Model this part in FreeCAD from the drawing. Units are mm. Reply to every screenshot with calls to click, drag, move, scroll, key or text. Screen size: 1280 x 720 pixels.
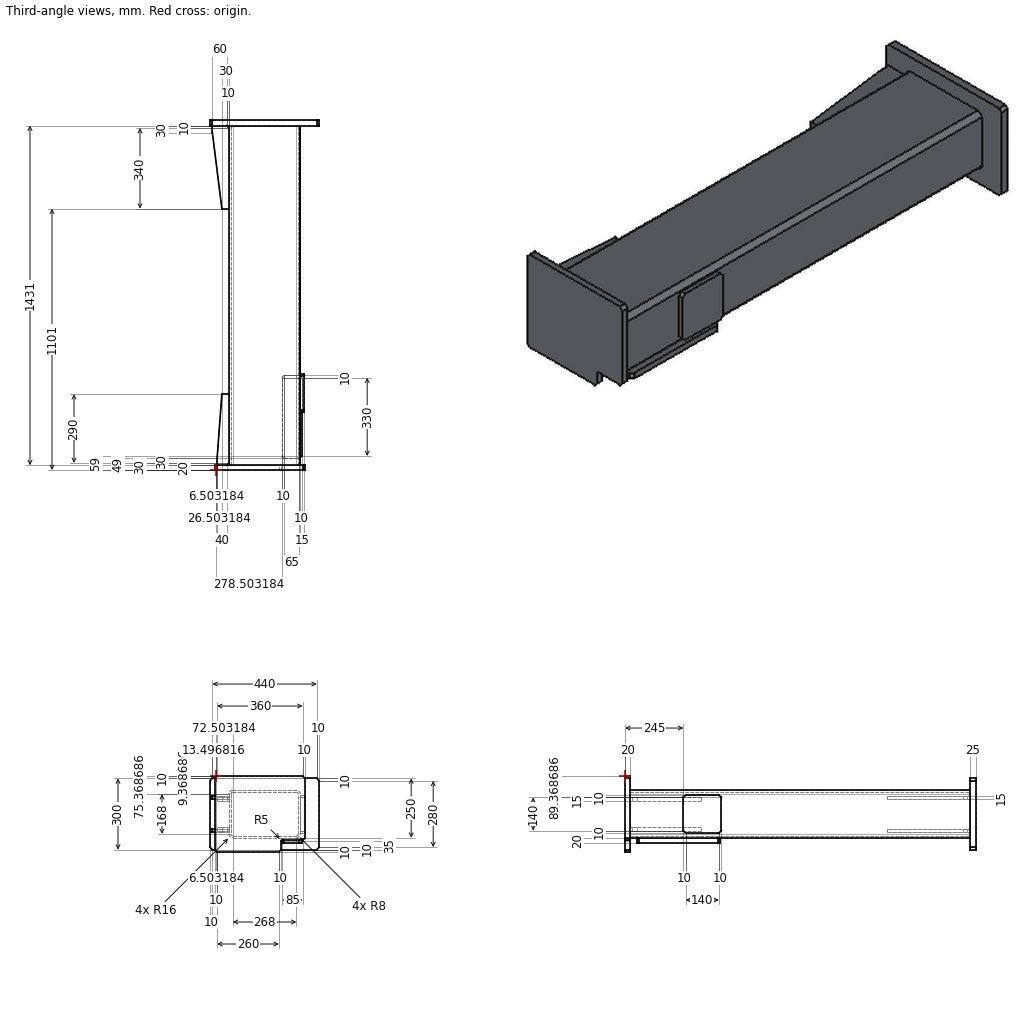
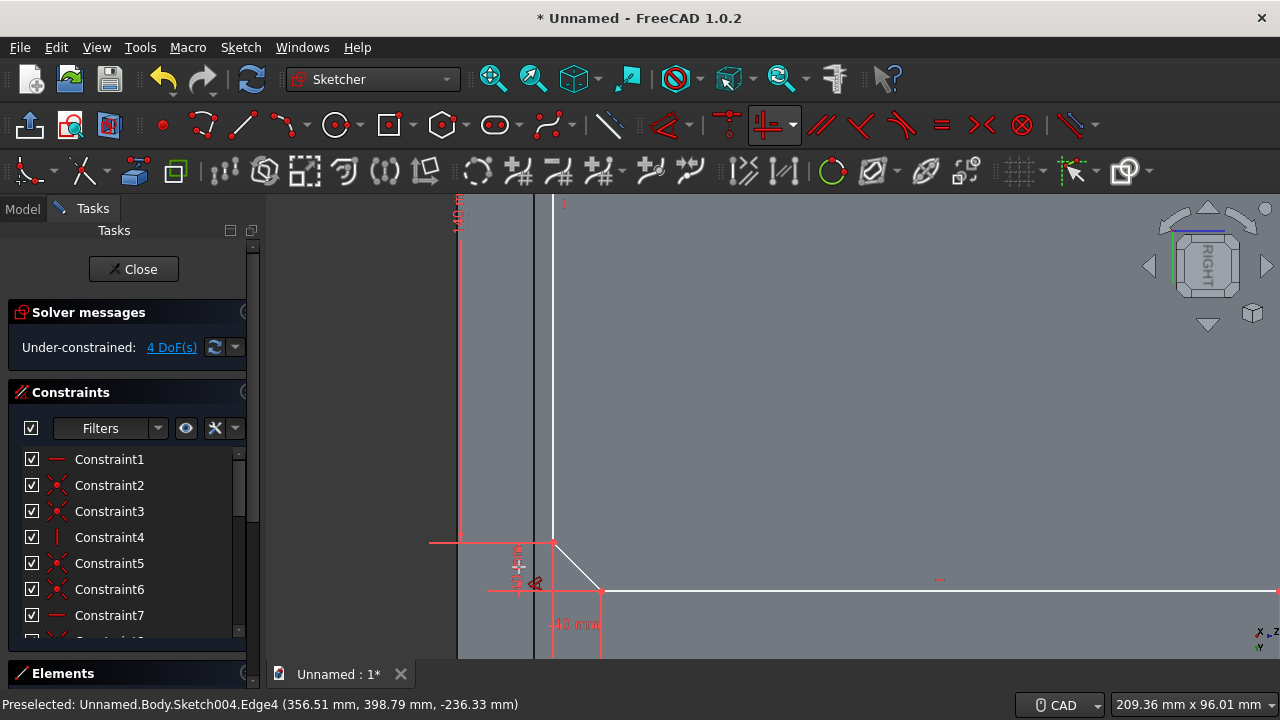
scroll(567, 558, down, 5)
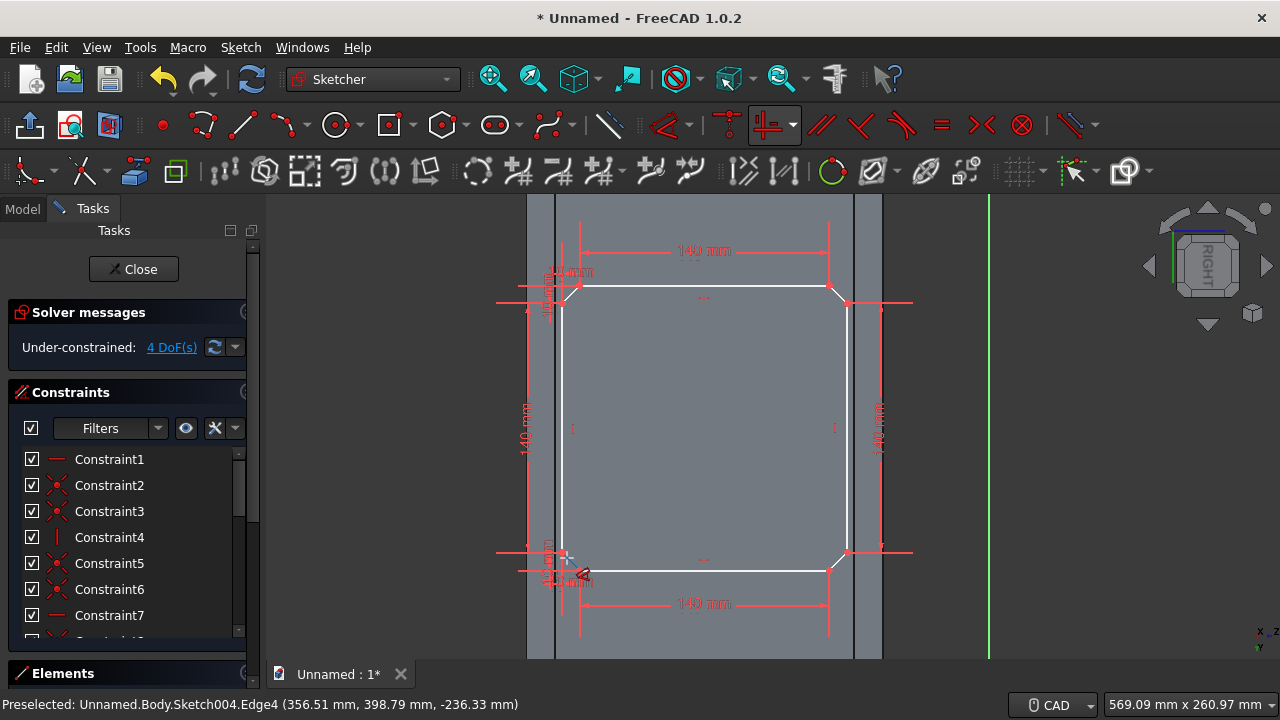
scroll(835, 565, up, 5)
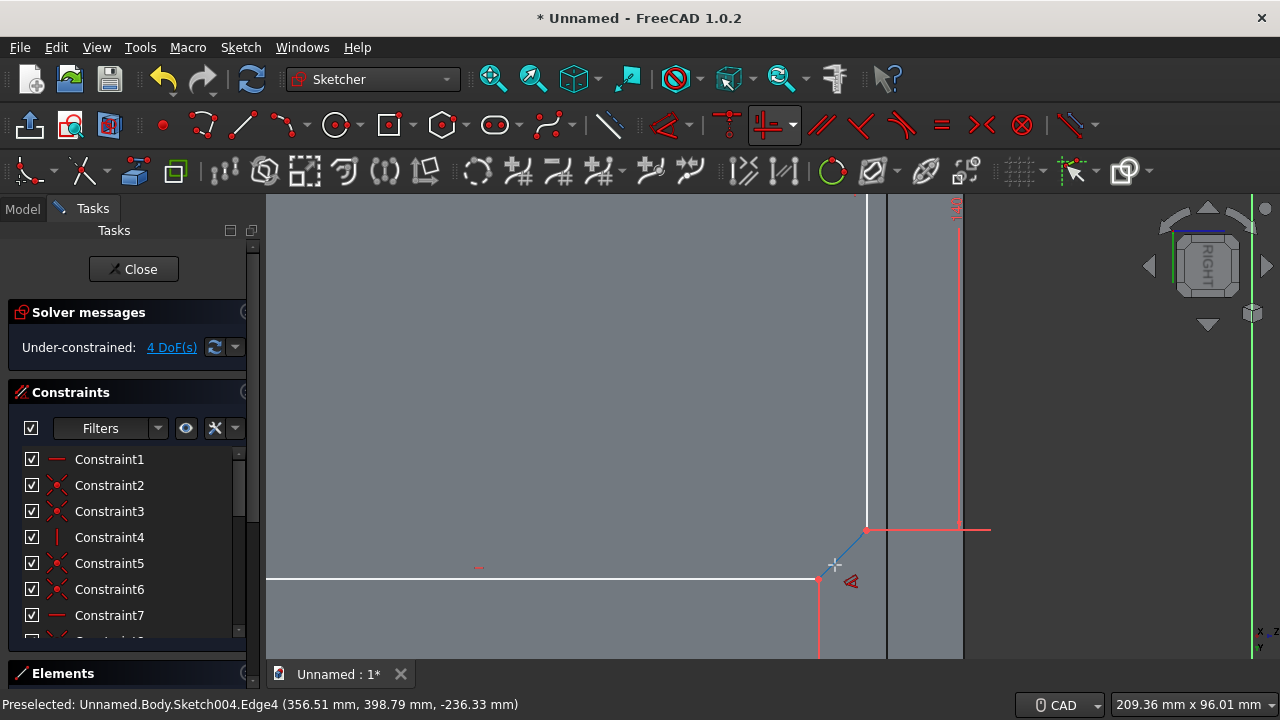
click(833, 564)
click(843, 613)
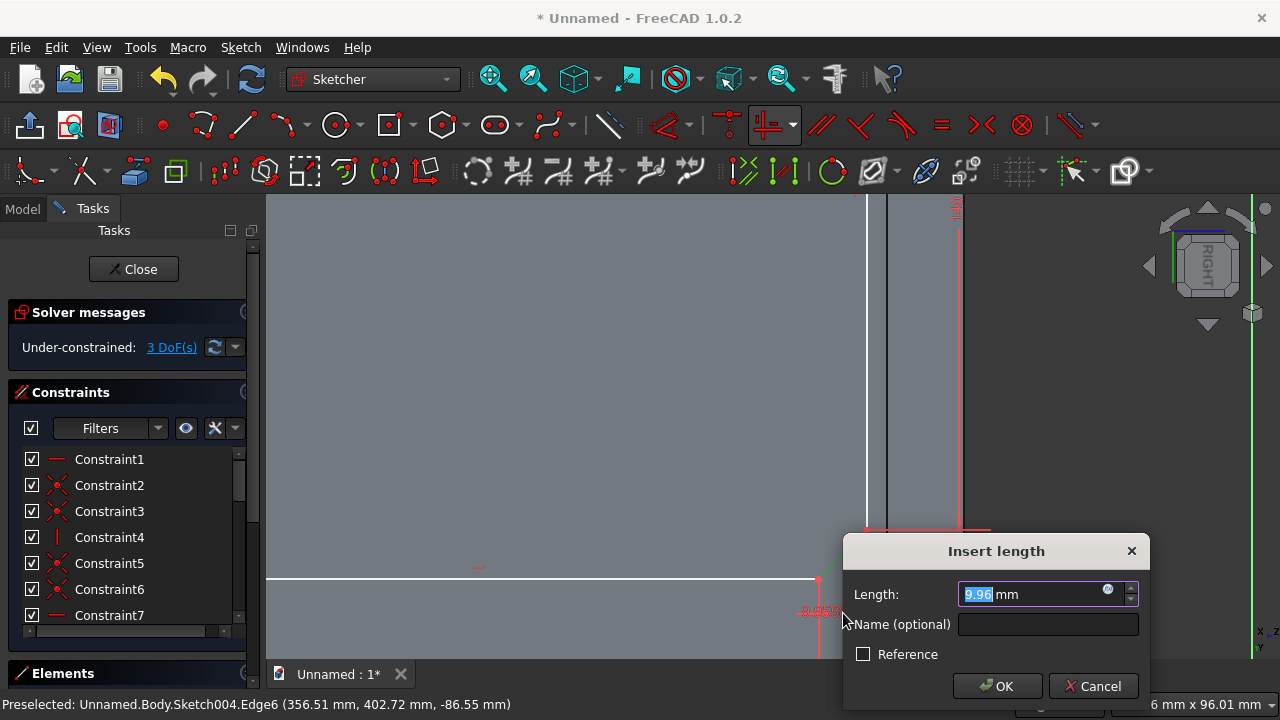
text(10)
key(Return)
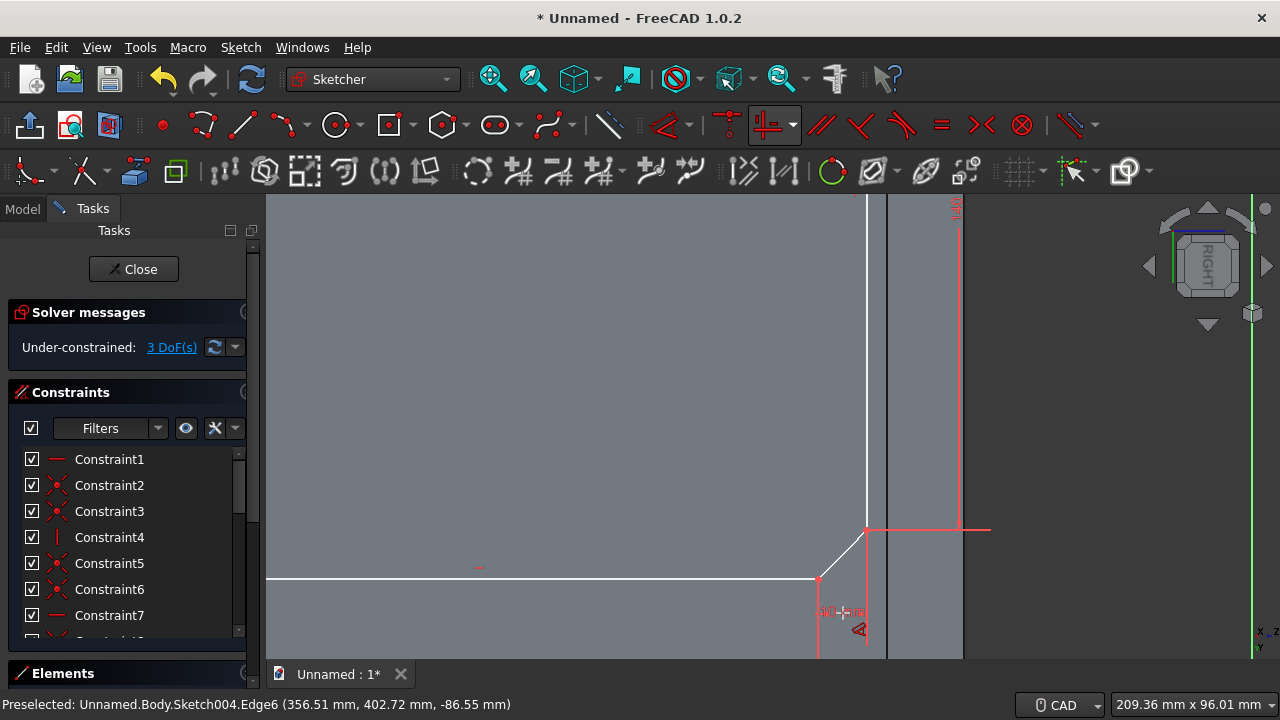
click(833, 564)
click(901, 555)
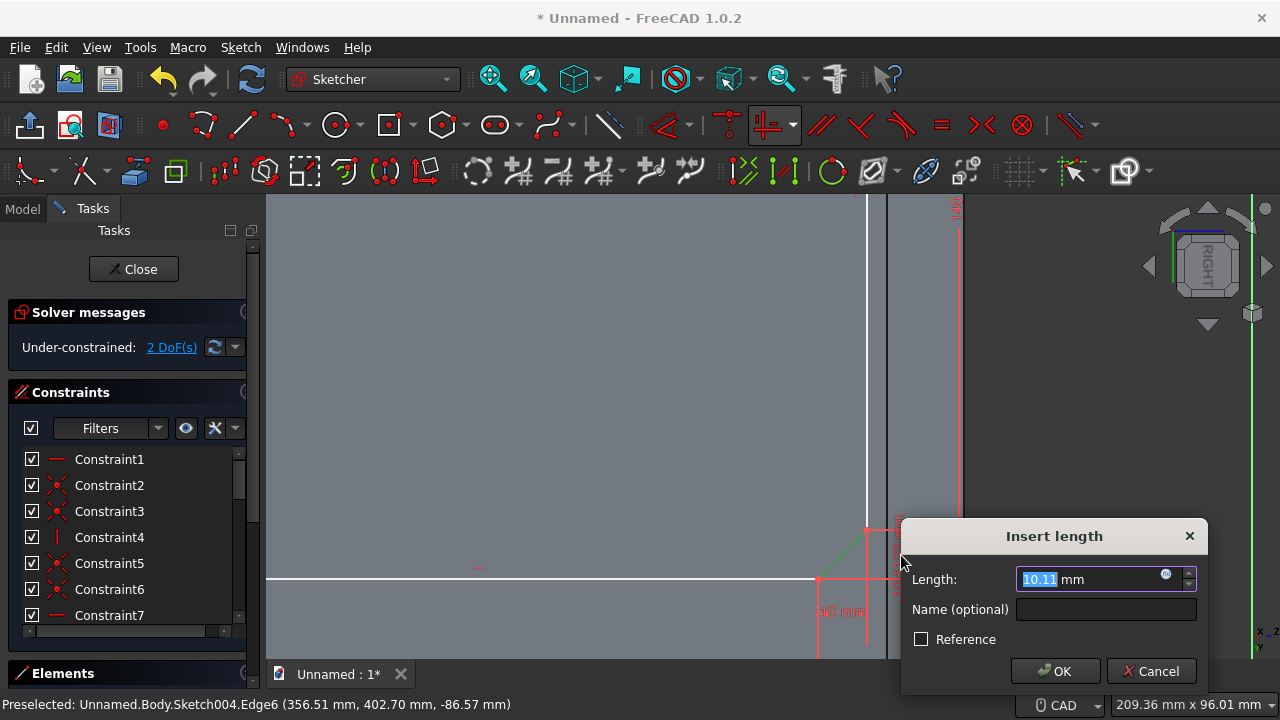
text(10)
key(Return)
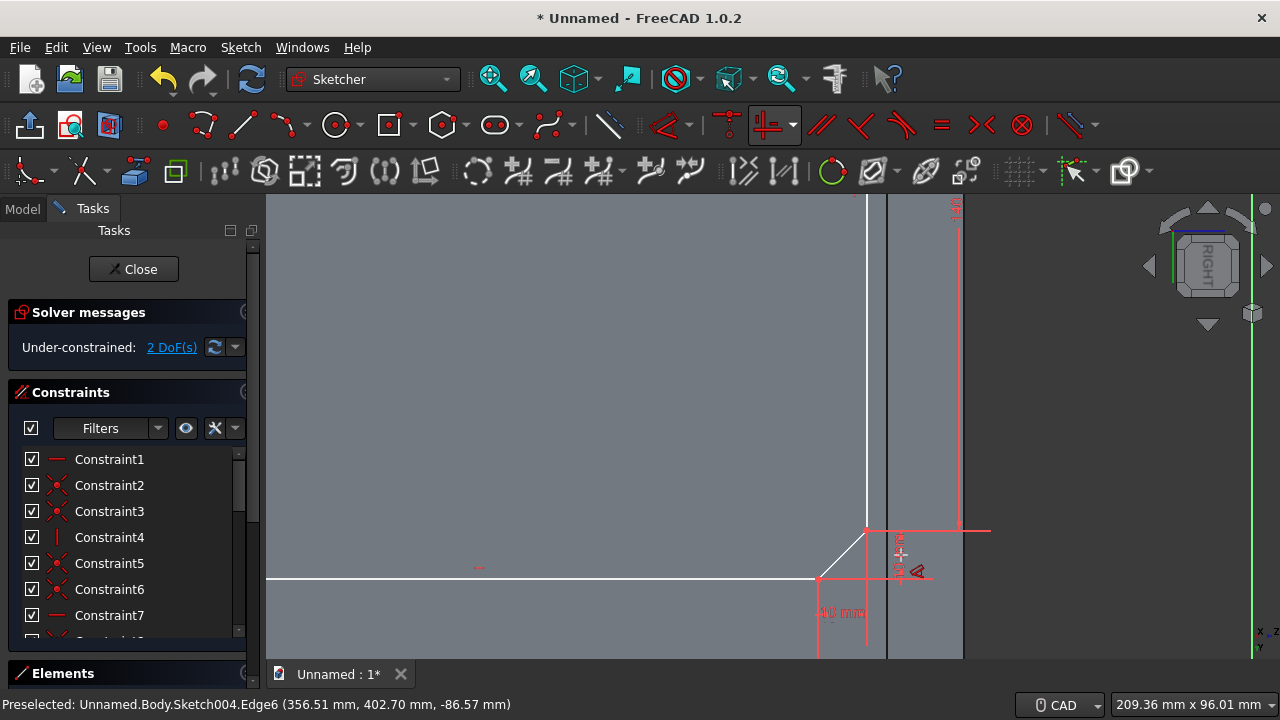
scroll(835, 565, down, 5)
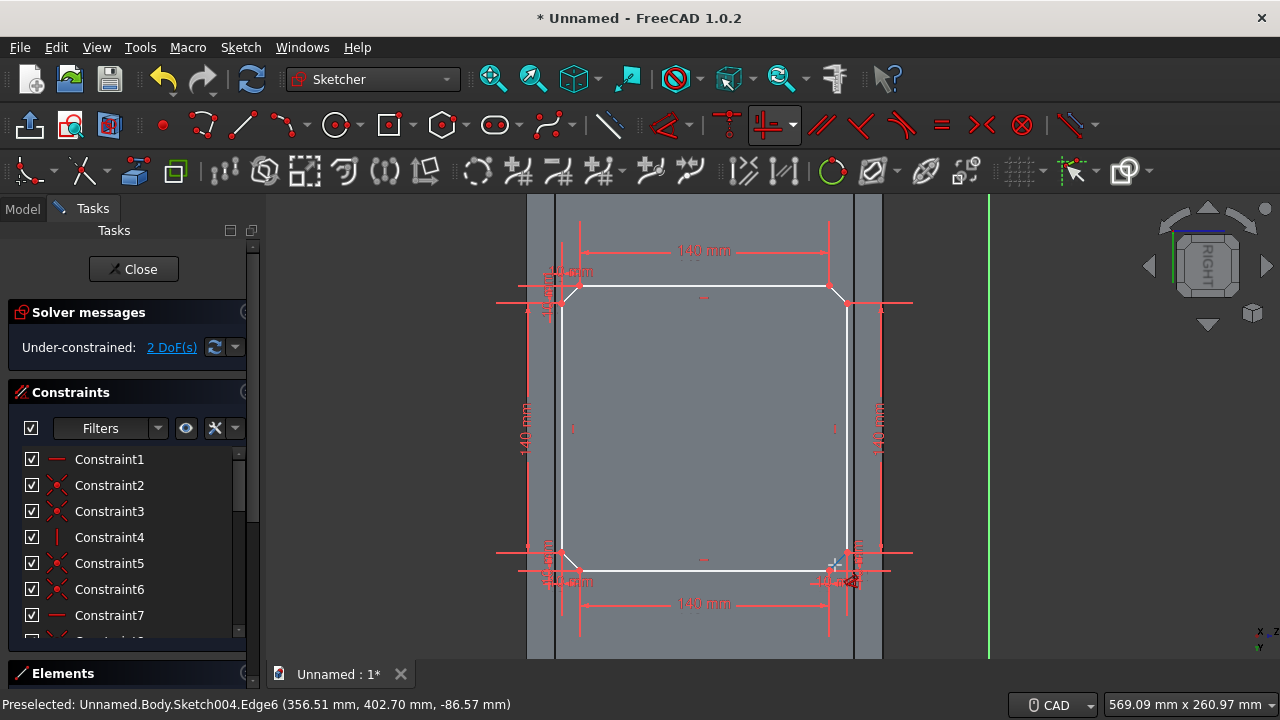
click(829, 286)
click(1023, 254)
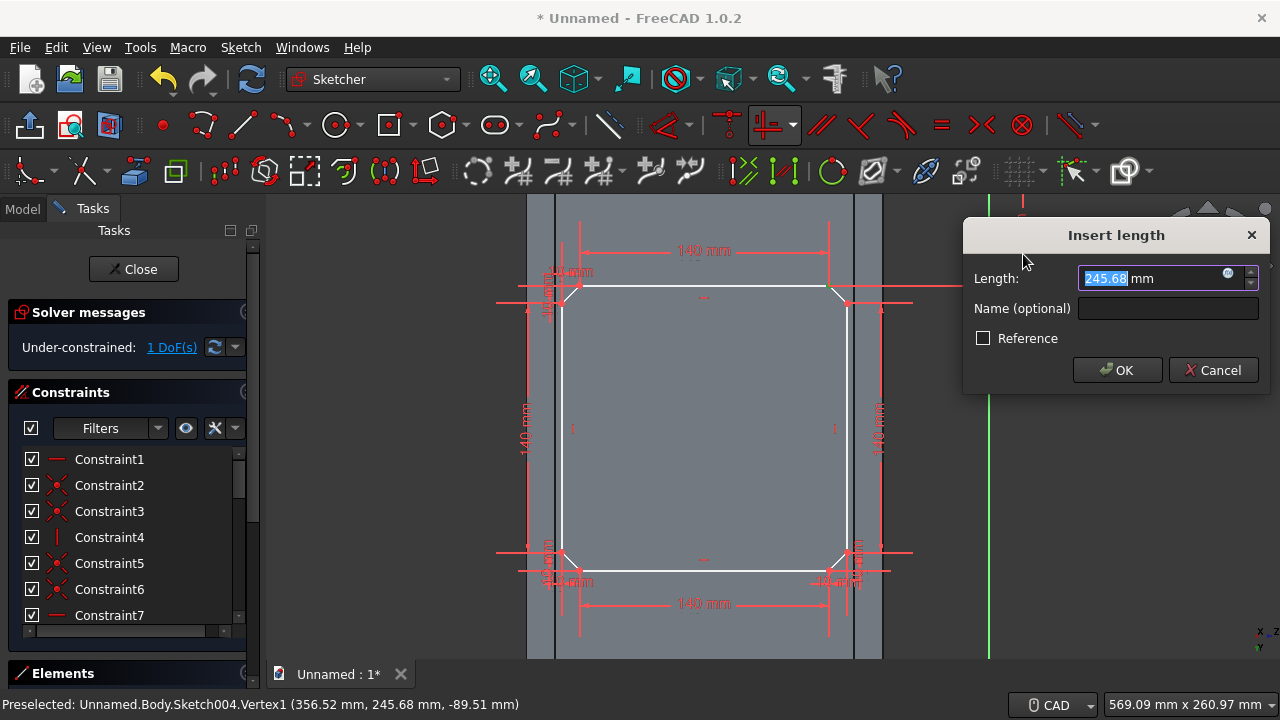
text(245)
key(Return)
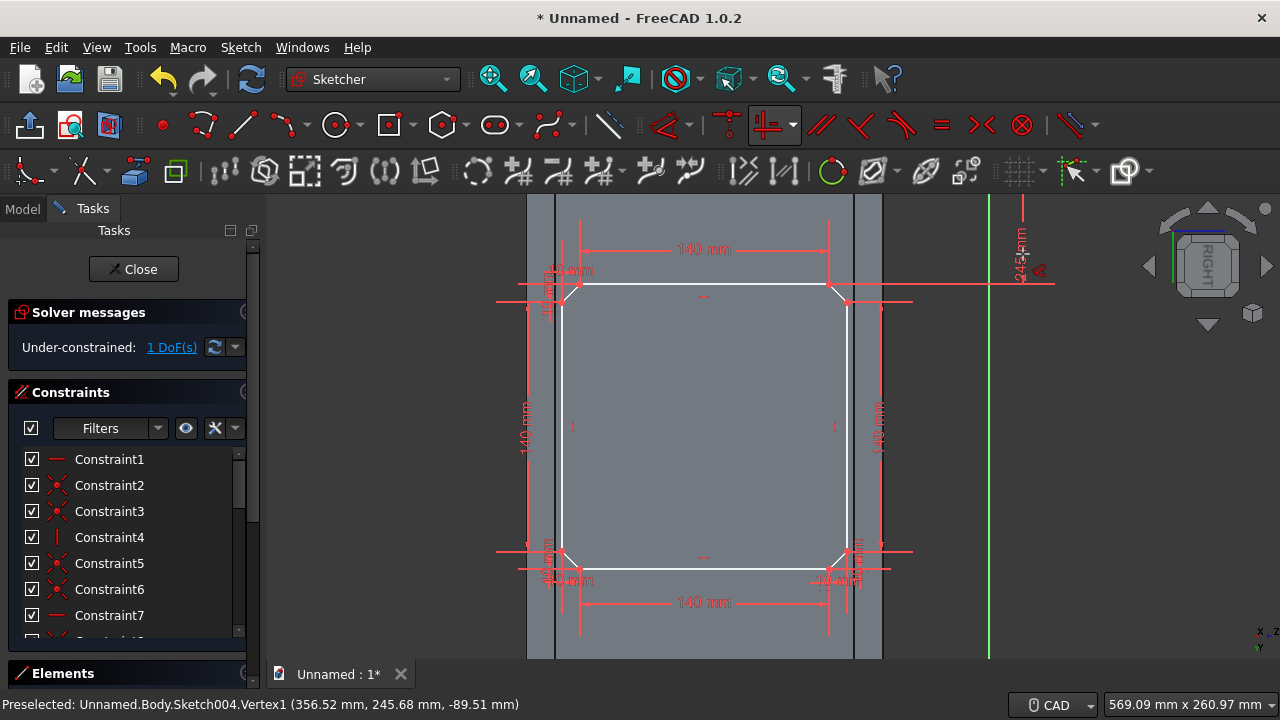
click(829, 284)
click(909, 318)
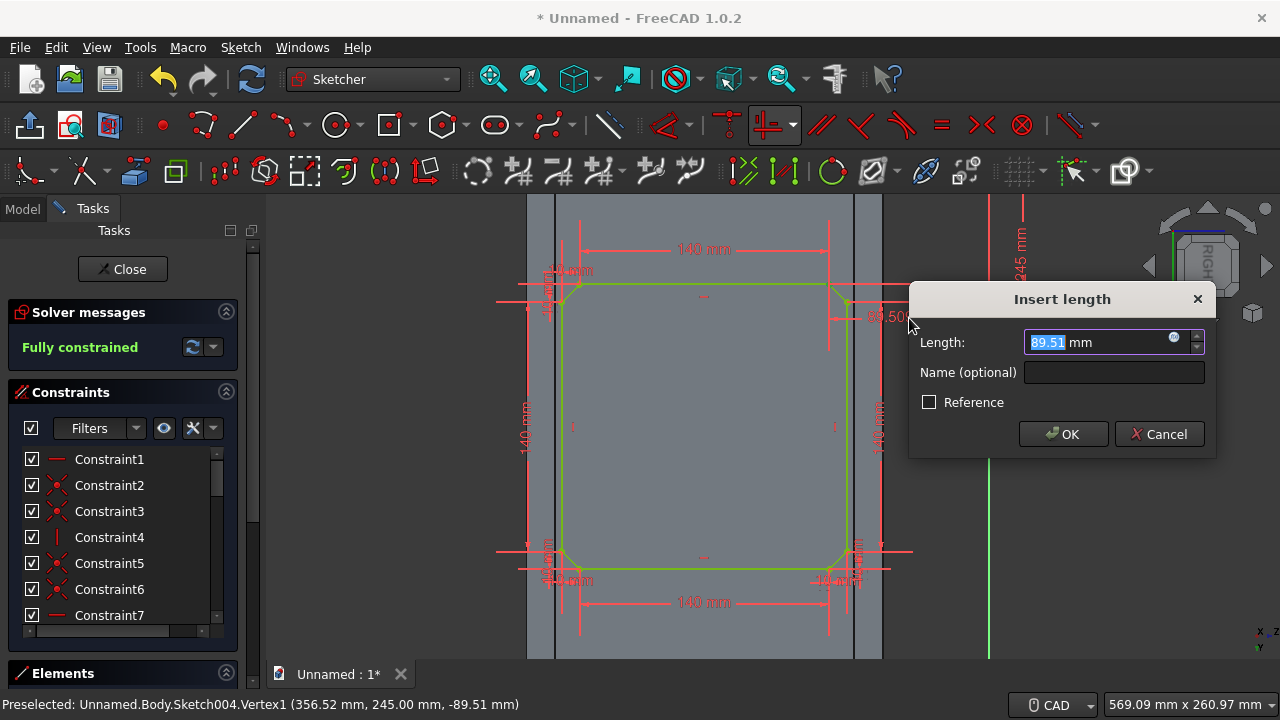
text(89.368686)
key(Return)
key(Escape)